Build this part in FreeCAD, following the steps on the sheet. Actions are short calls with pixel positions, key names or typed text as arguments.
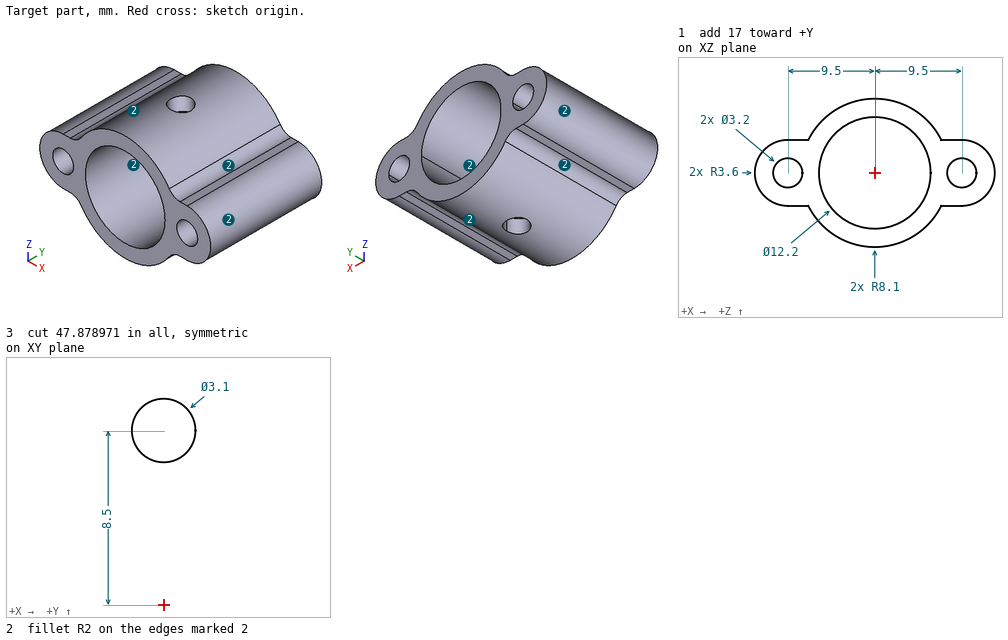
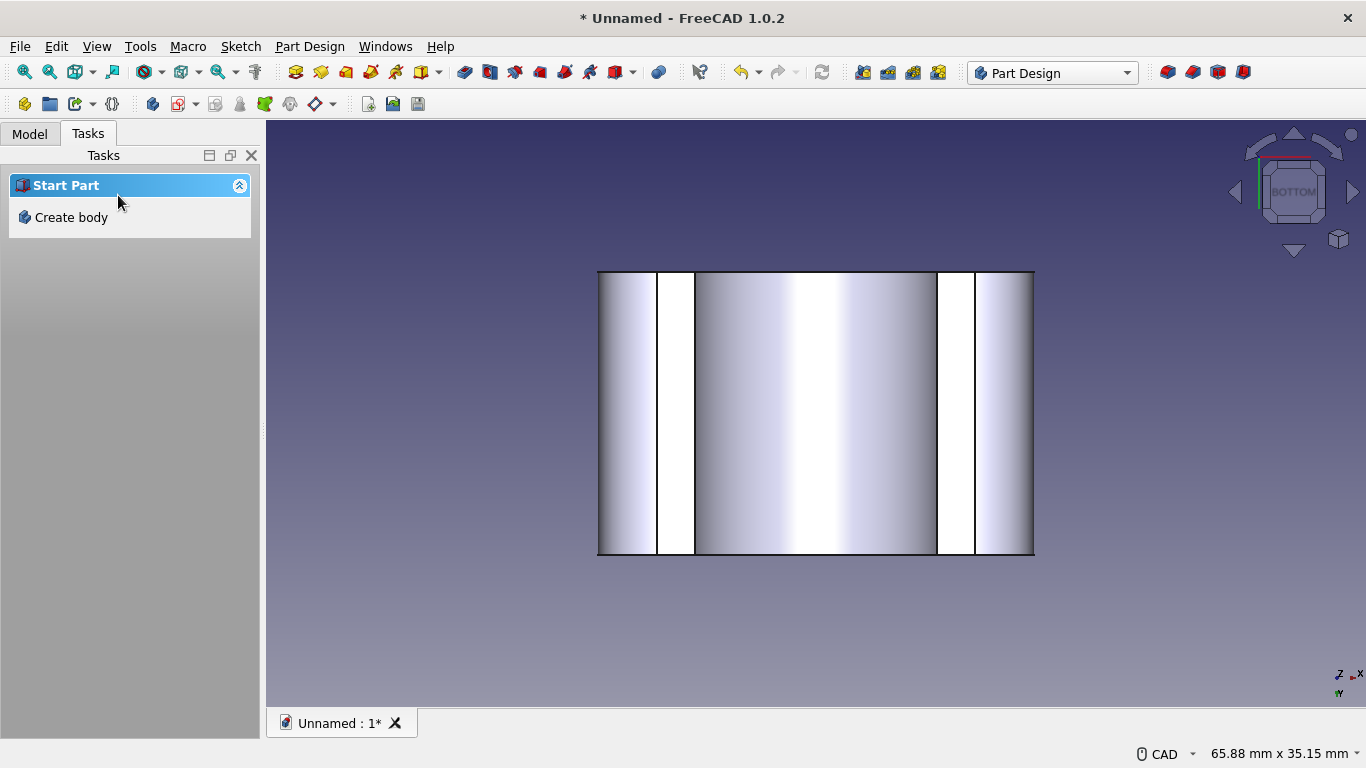
key(4)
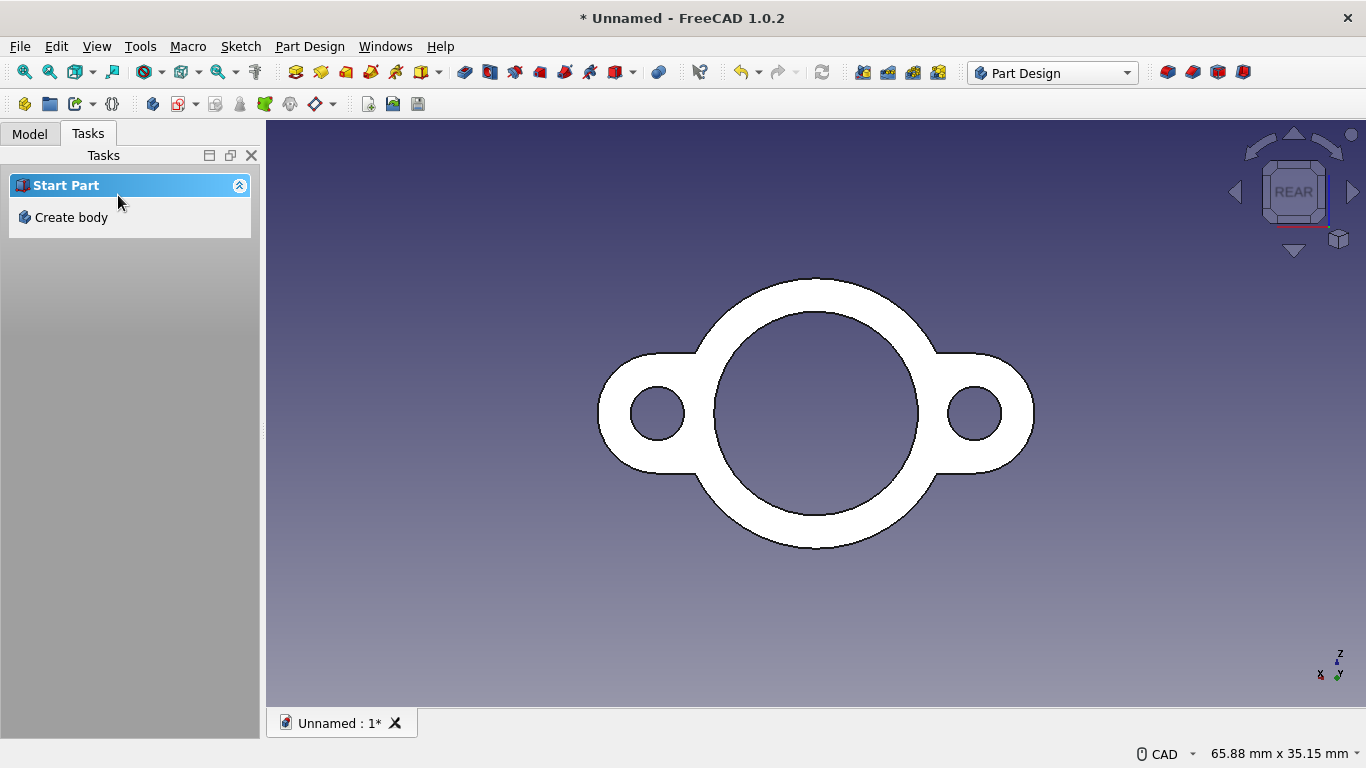
key(6)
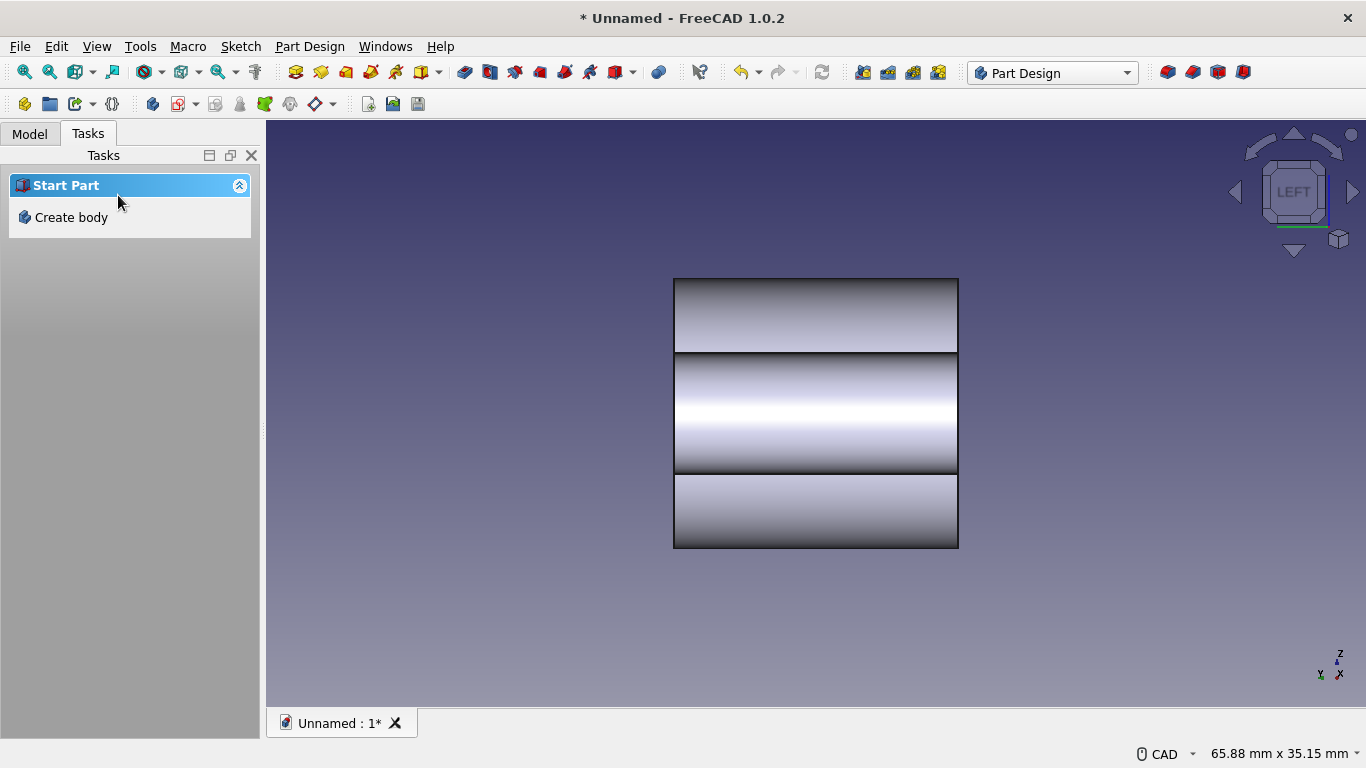
key(v)
key(3)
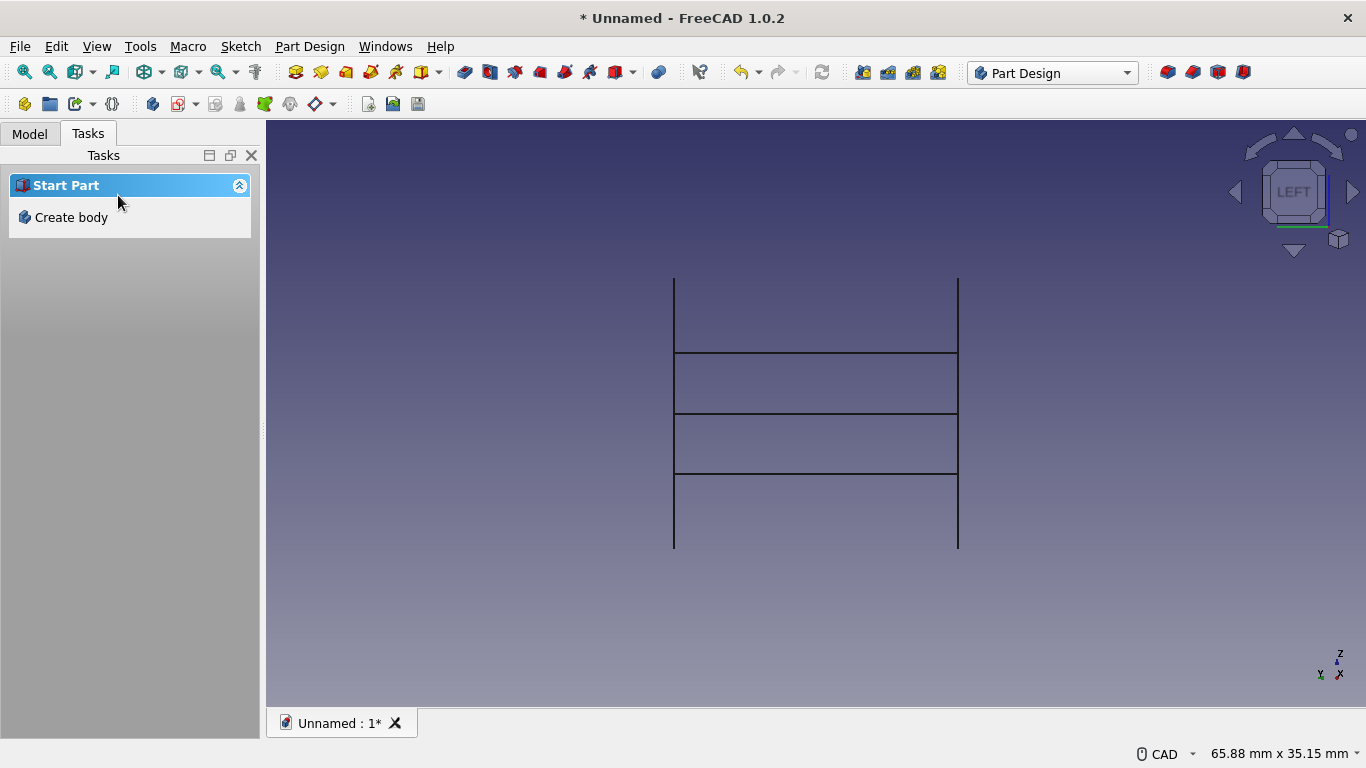
key(0)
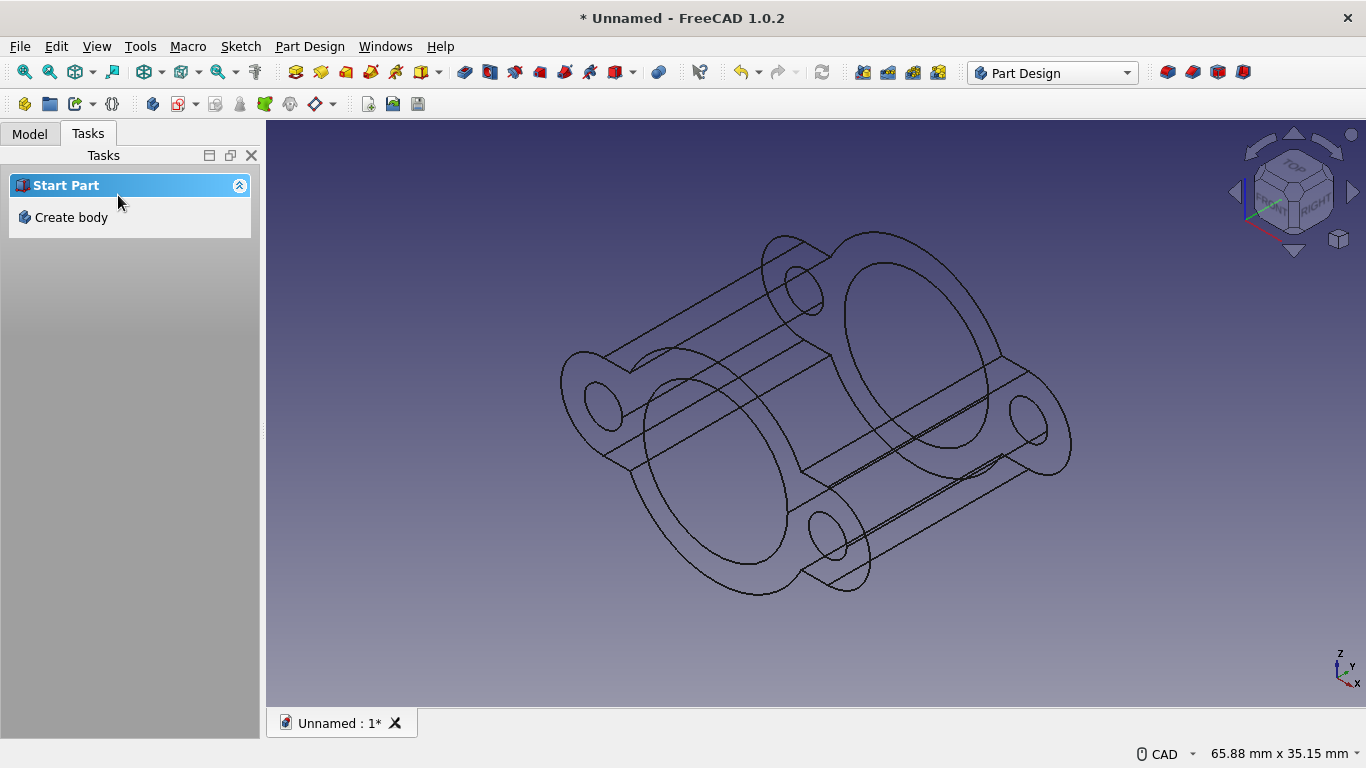
click(730, 412)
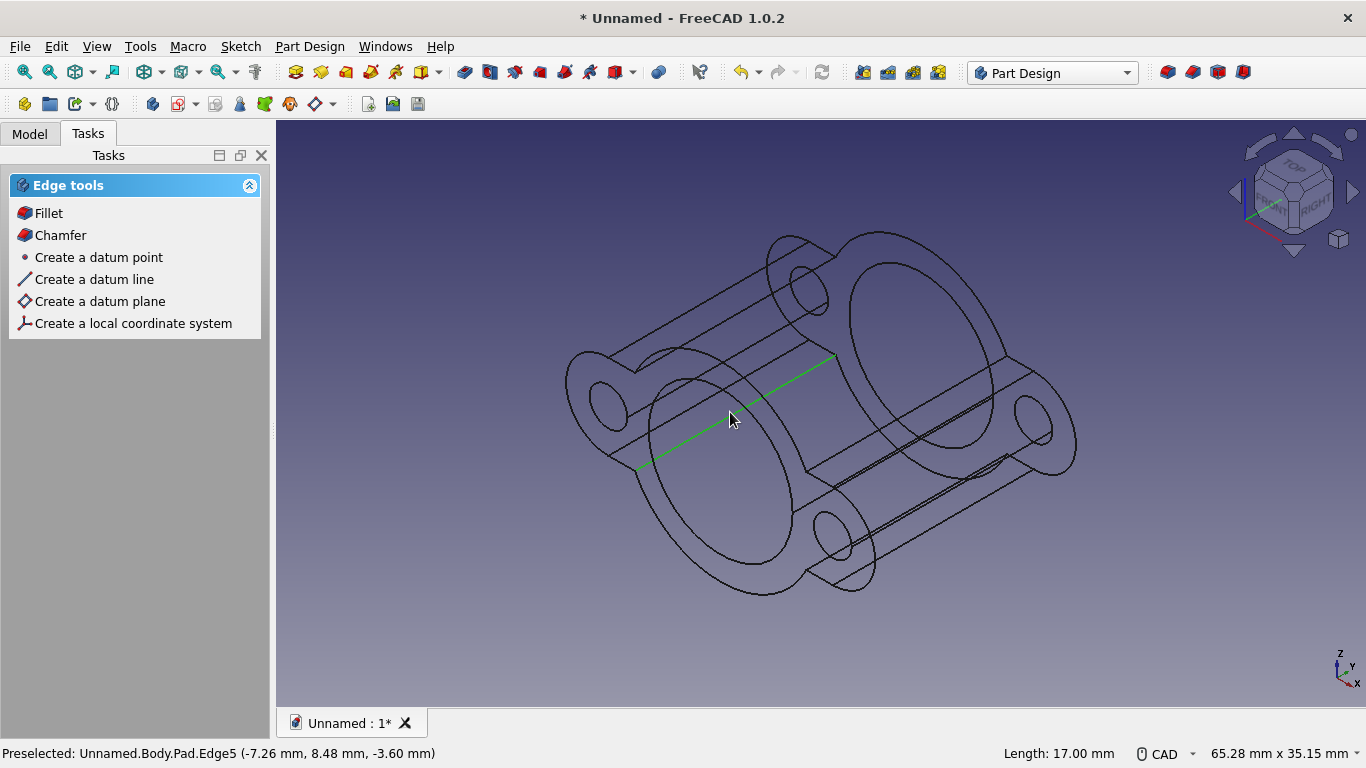
click(907, 413, ctrl)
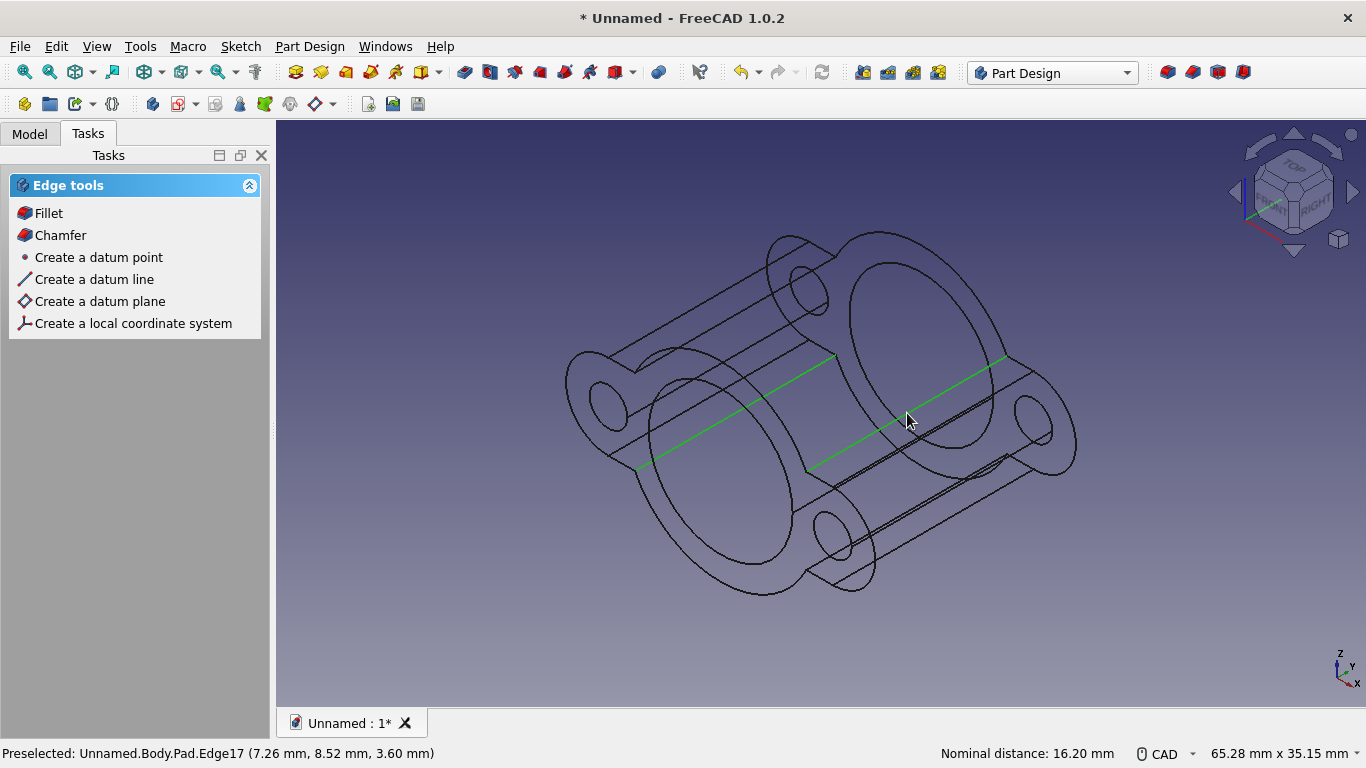
click(735, 314, ctrl)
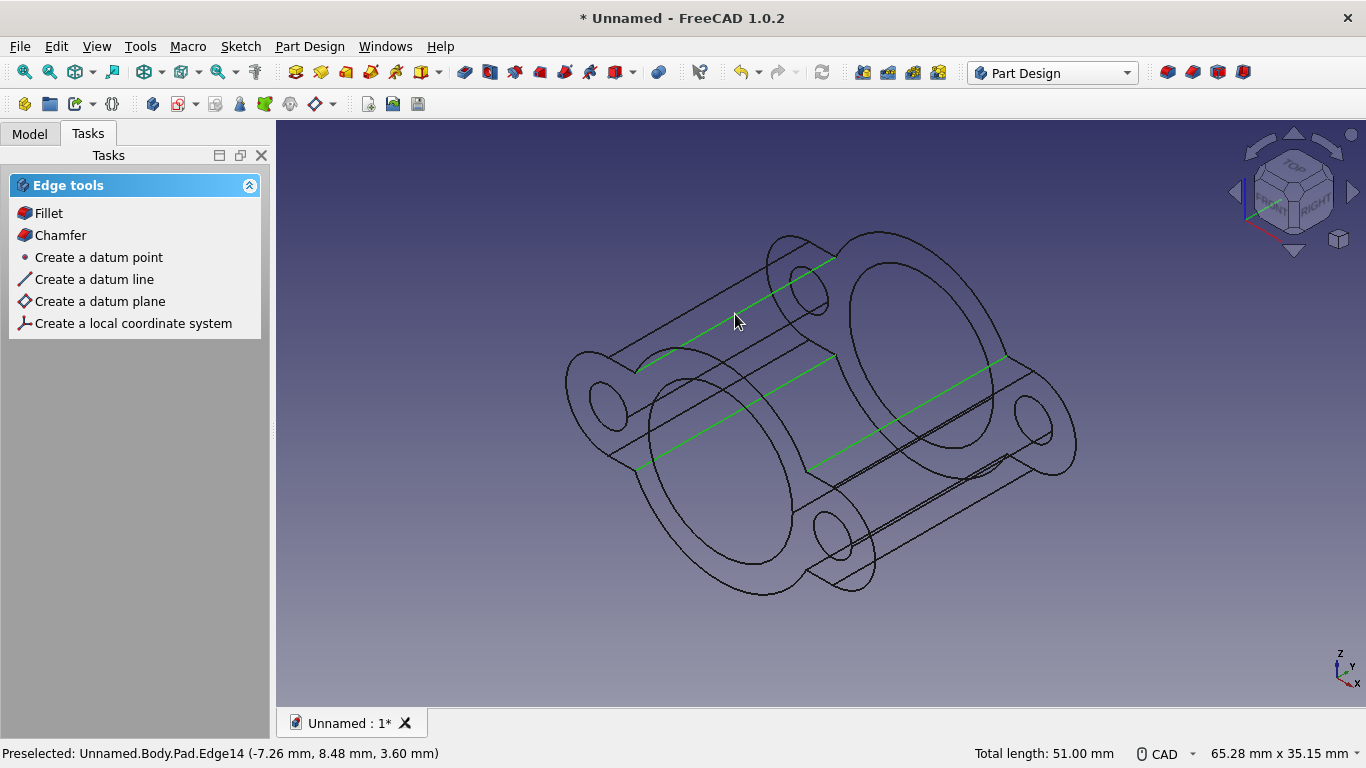
scroll(907, 511, up, 6)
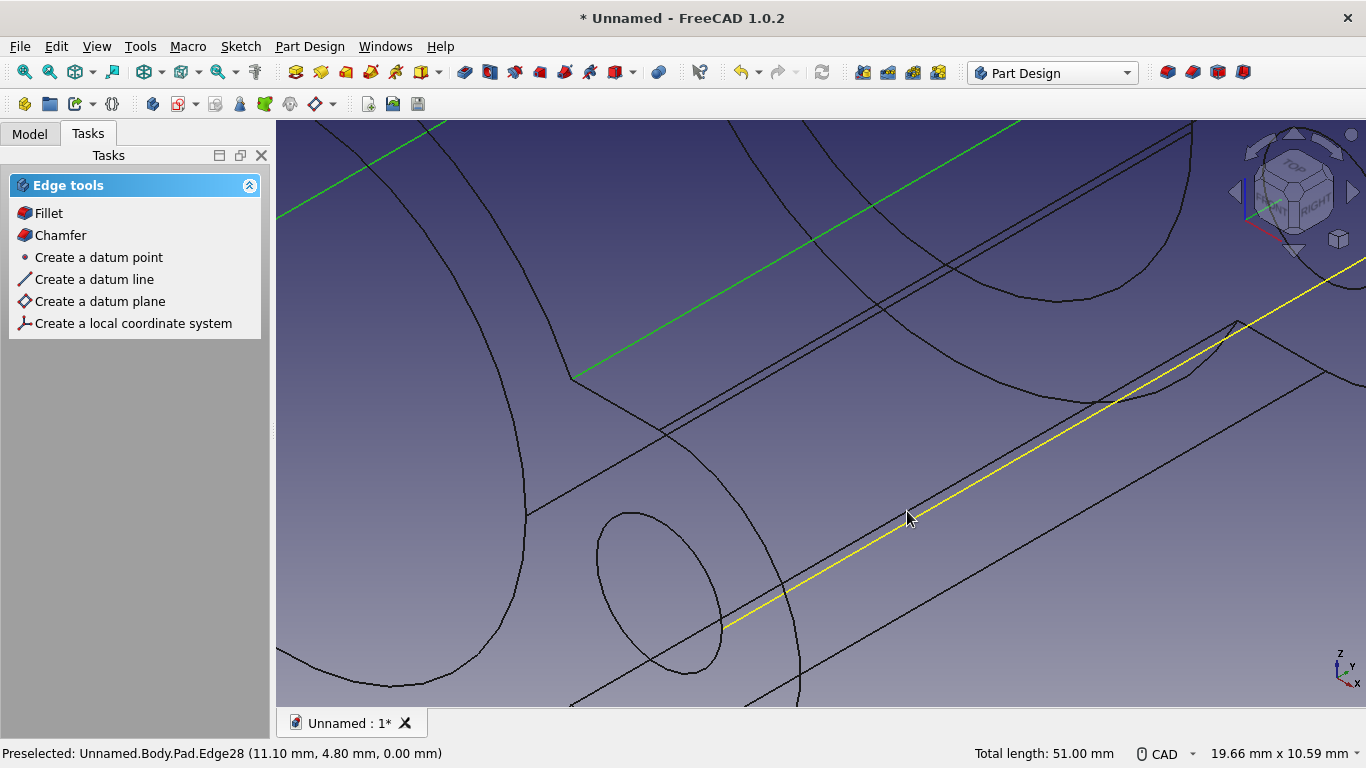
click(905, 512, ctrl)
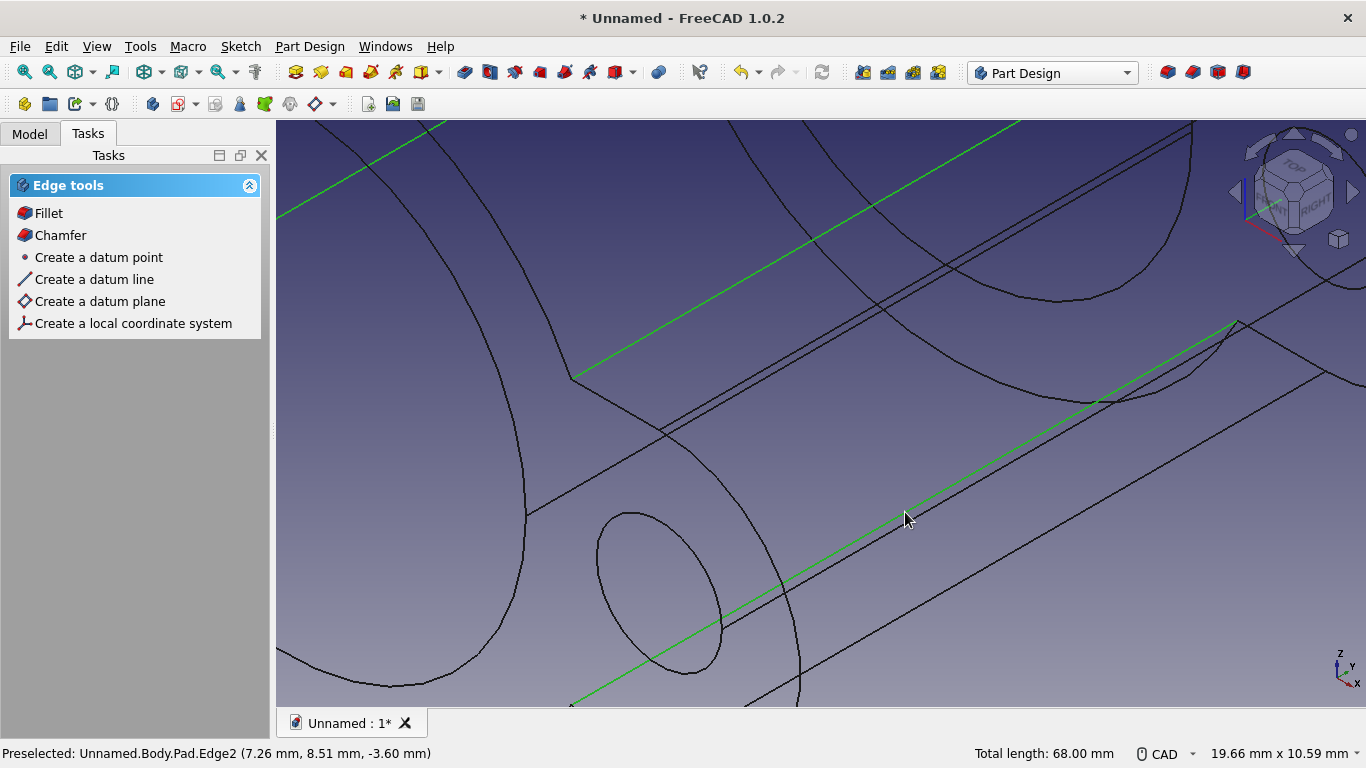
key(v)
key(1)